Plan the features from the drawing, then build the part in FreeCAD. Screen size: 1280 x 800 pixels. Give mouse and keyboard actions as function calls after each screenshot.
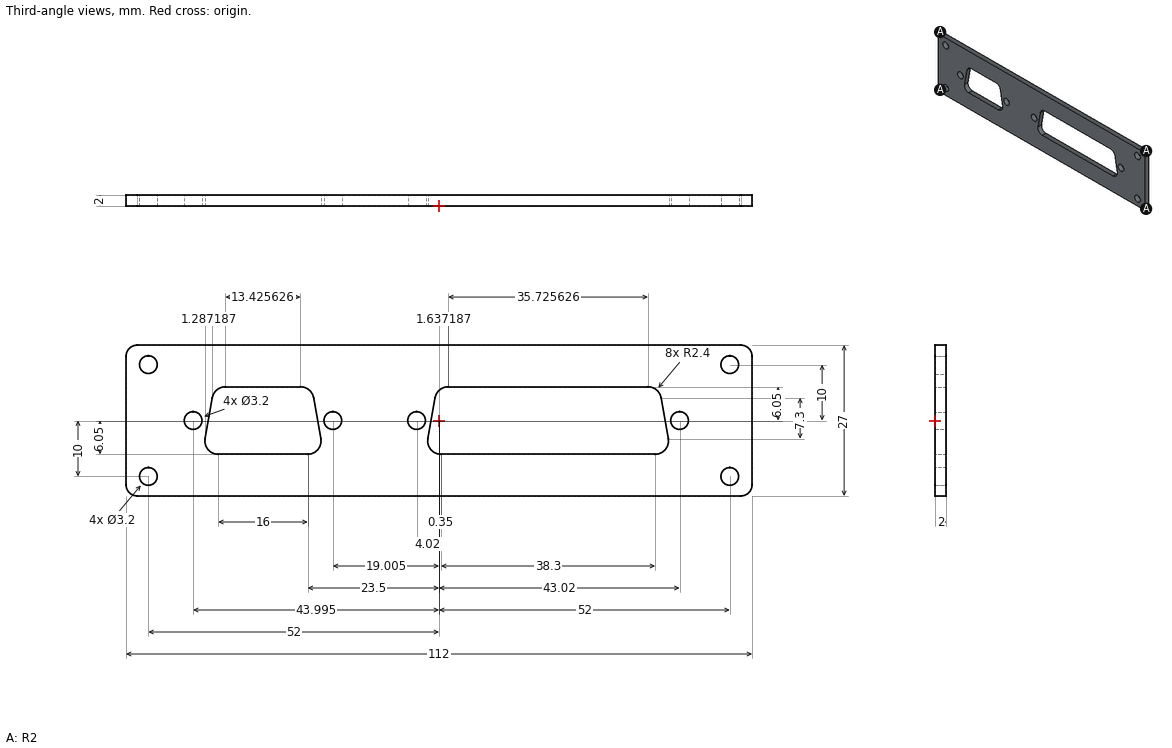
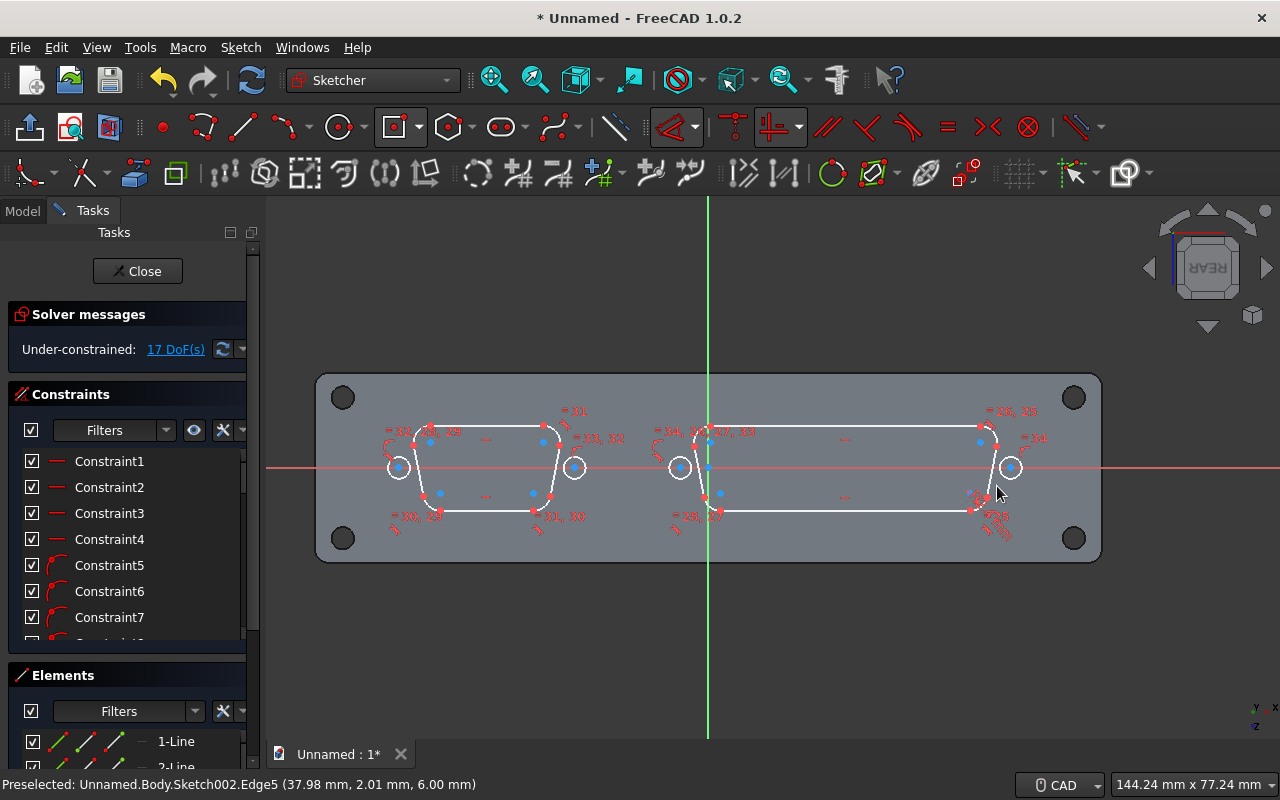
scroll(407, 460, up, 3)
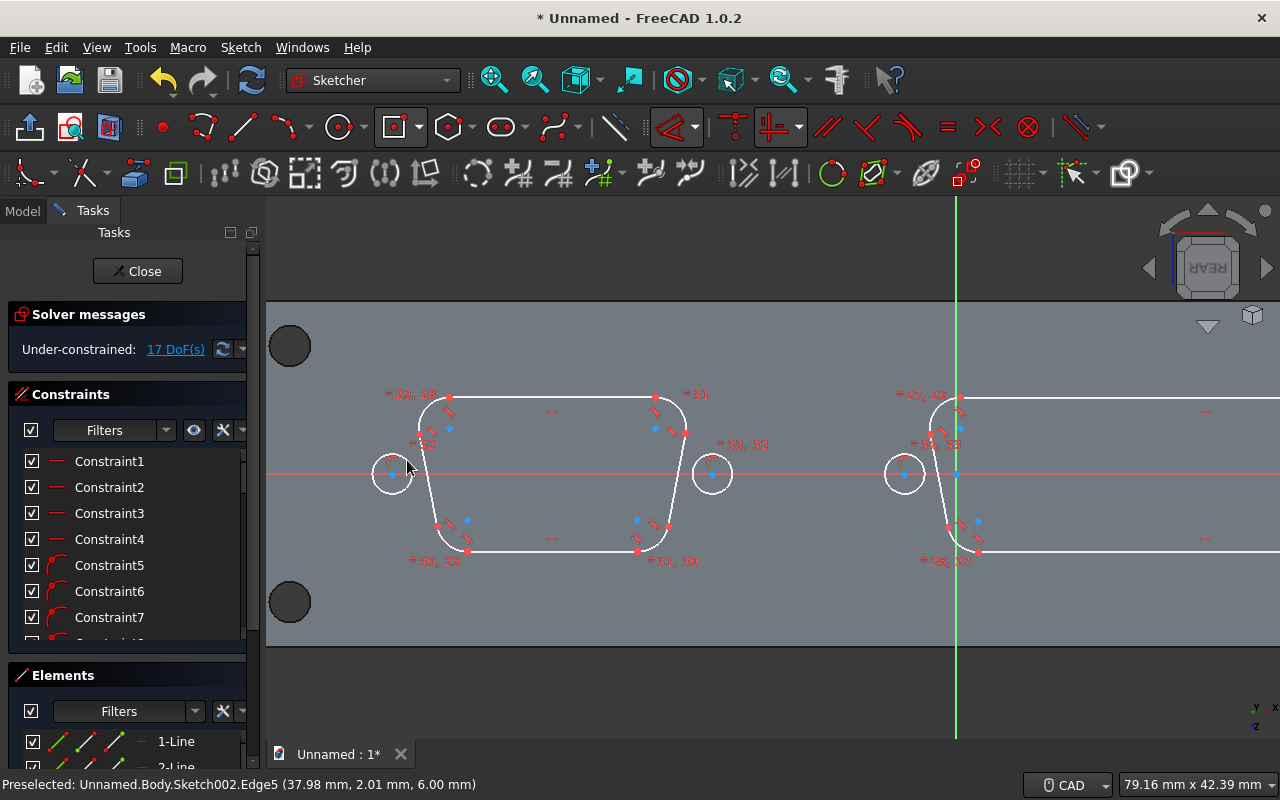
click(406, 460)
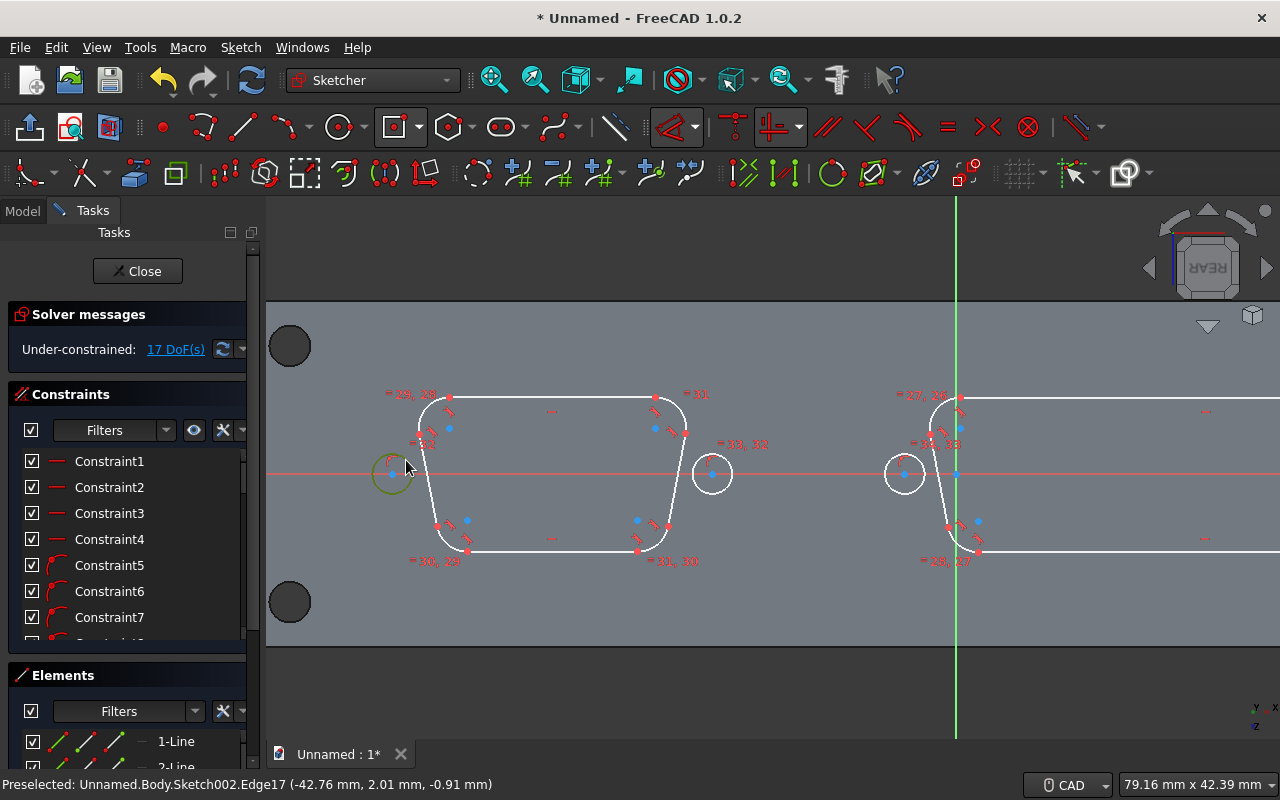
key(k)
key(o)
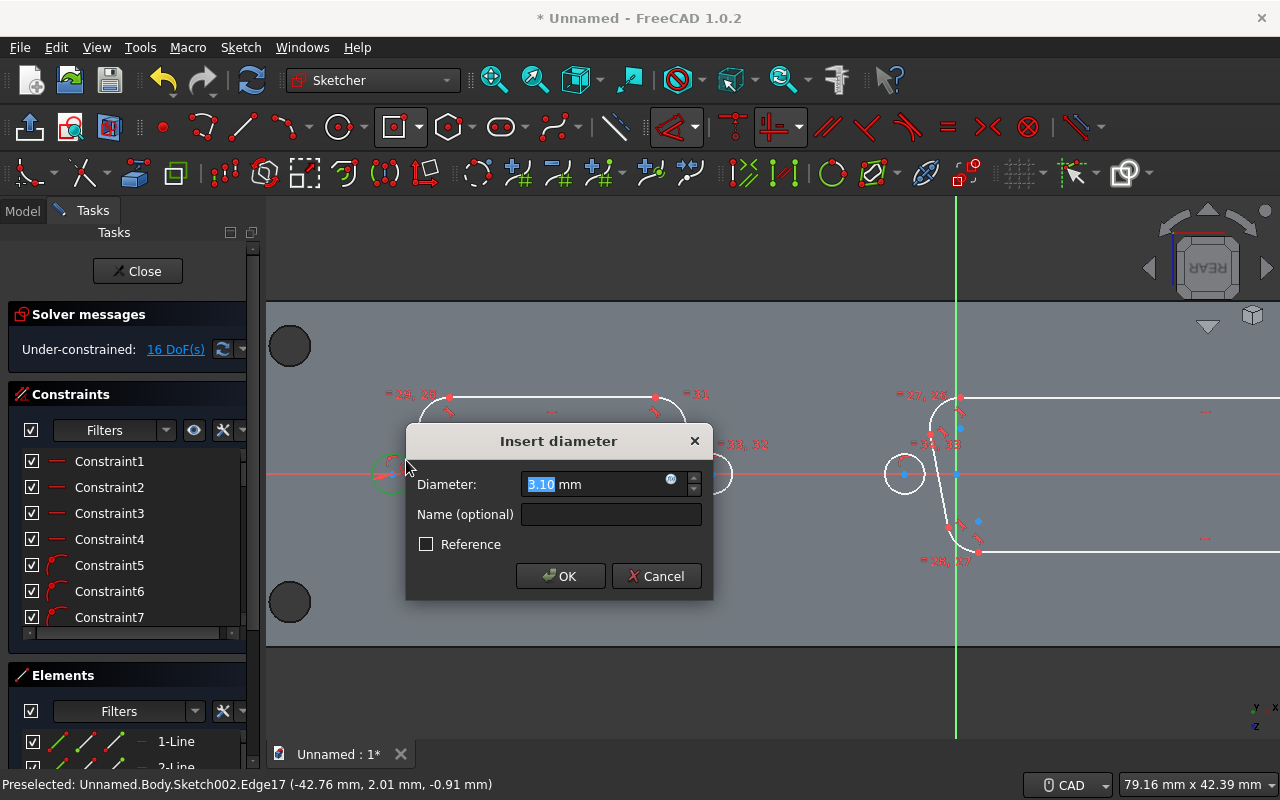
text(3.2)
key(Return)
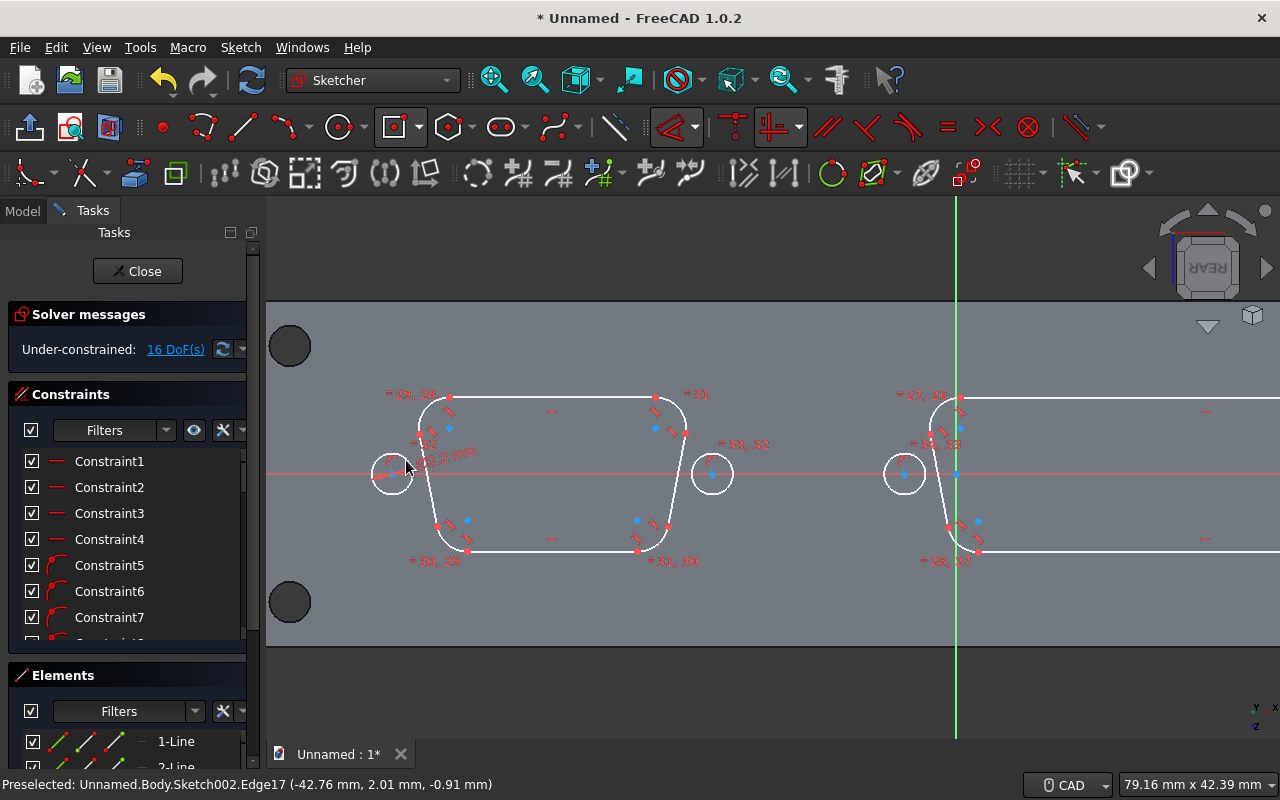
click(594, 397)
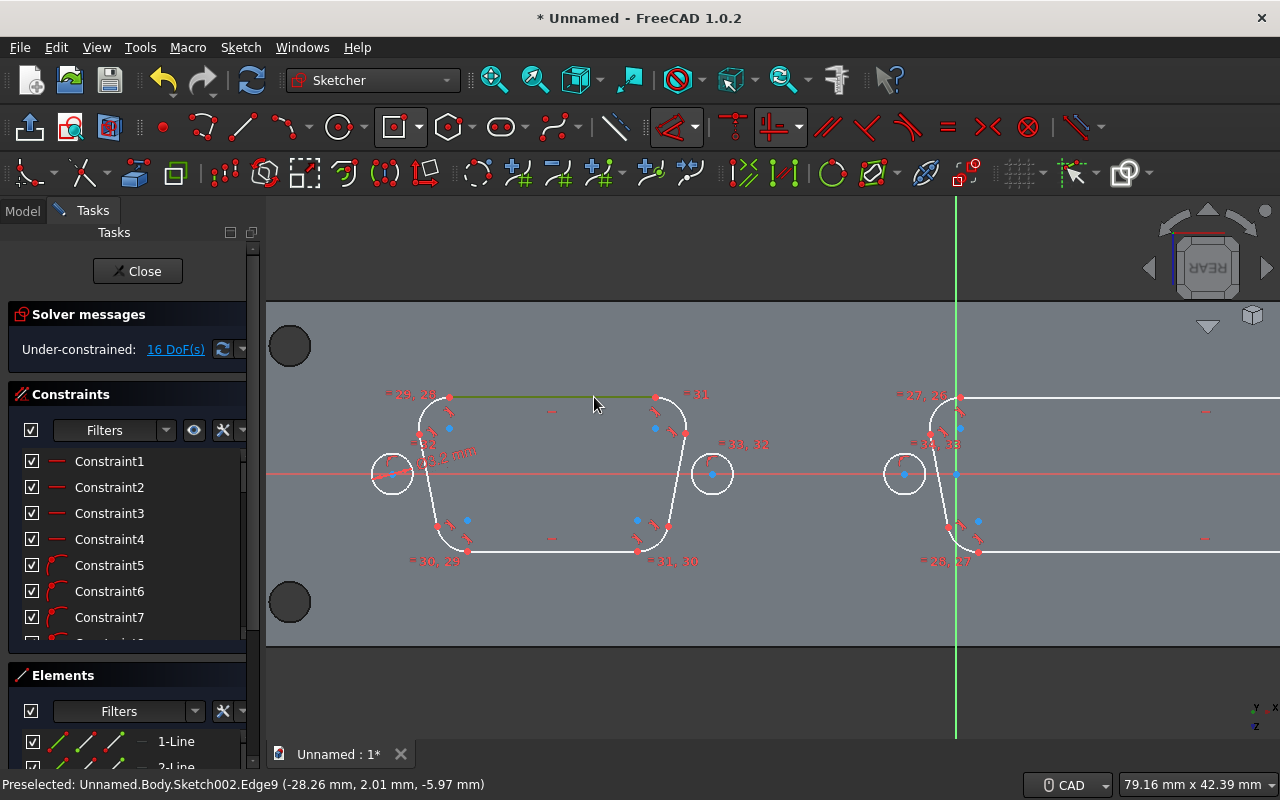
click(698, 128)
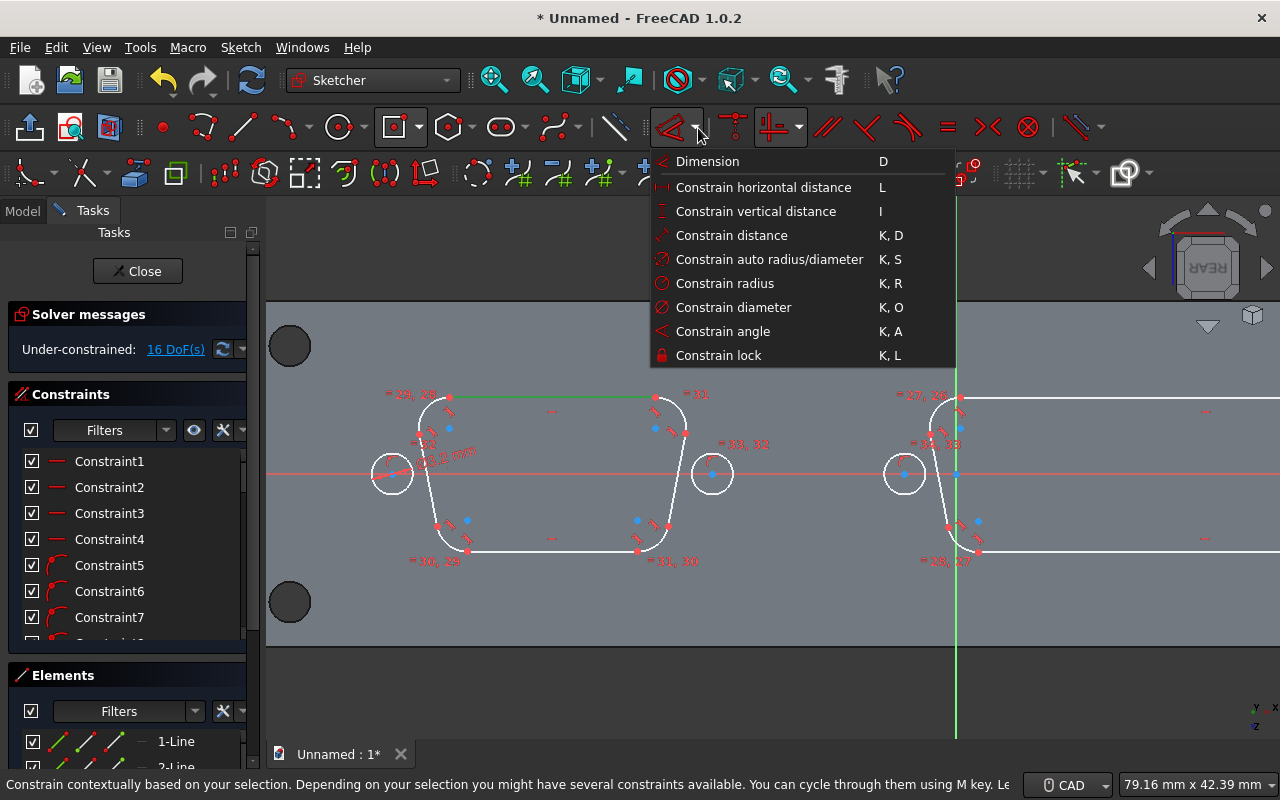
click(803, 187)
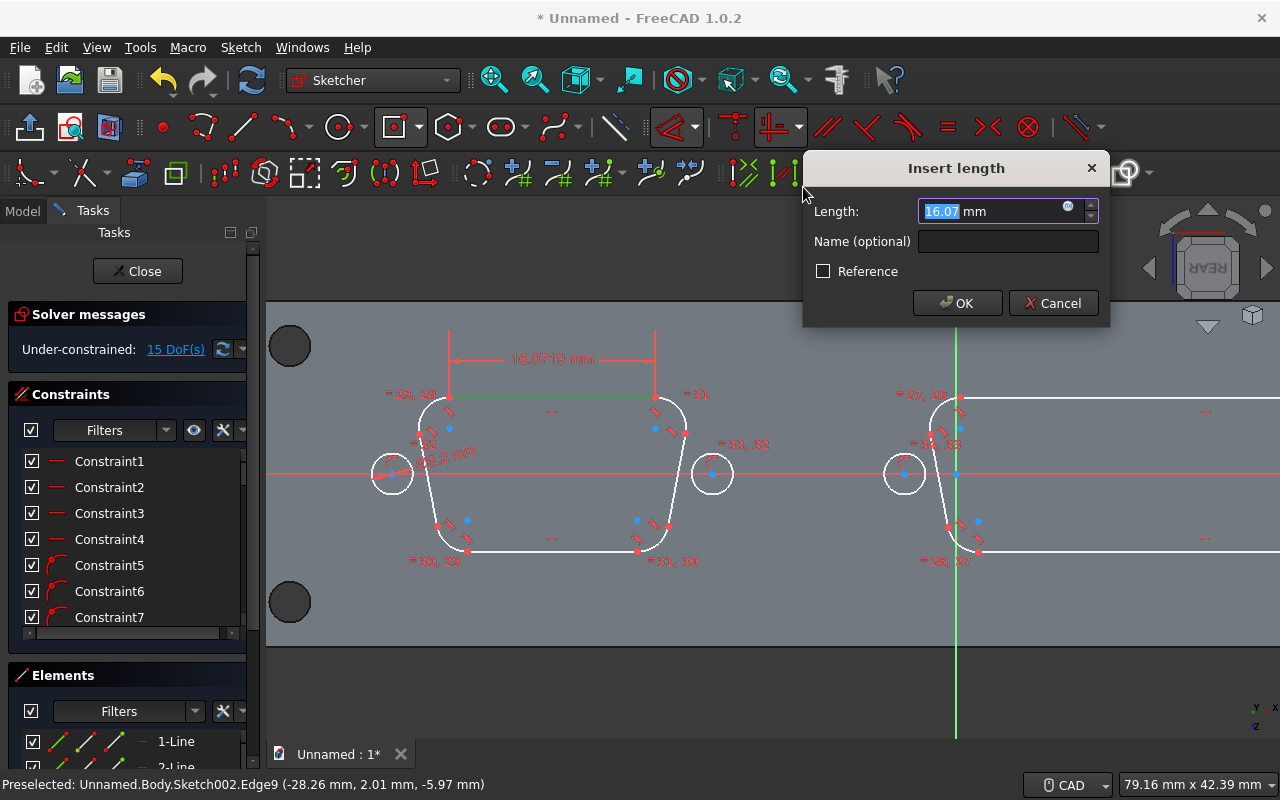
text(16)
key(Return)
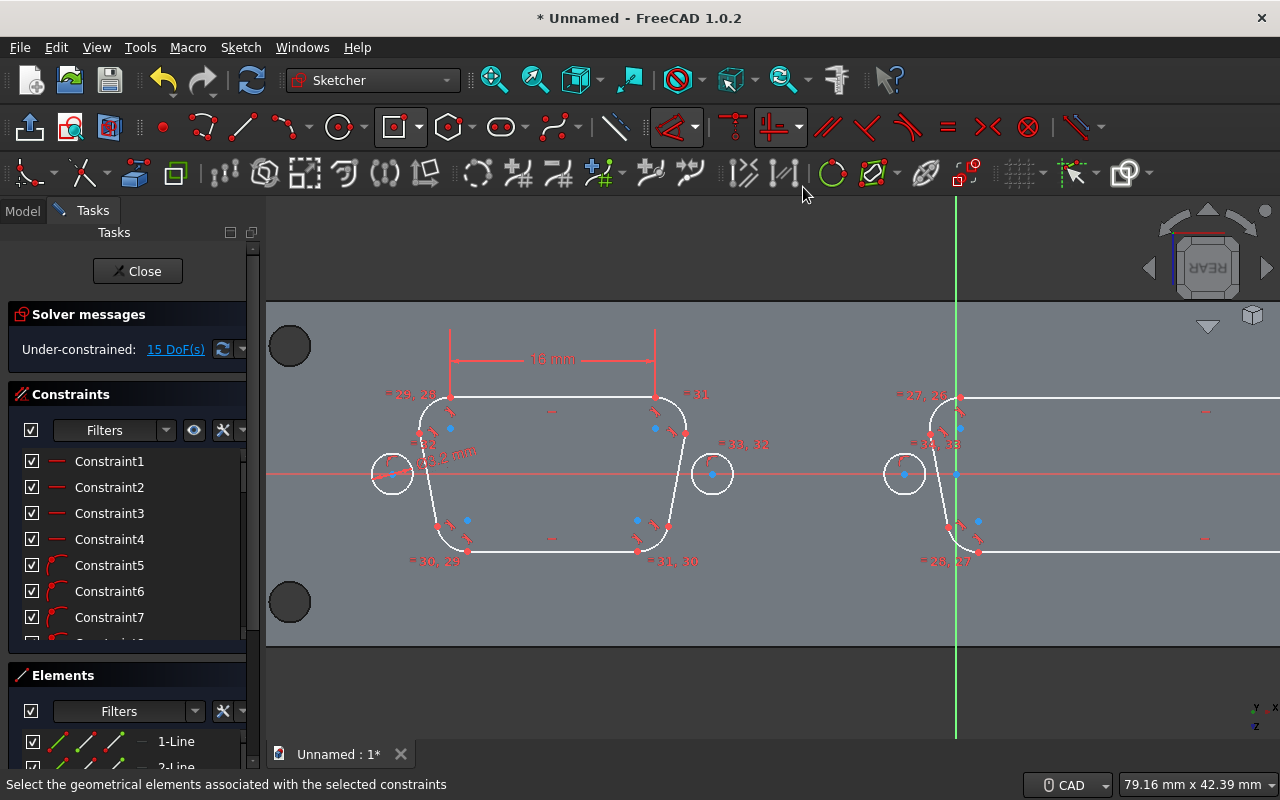
click(1108, 398)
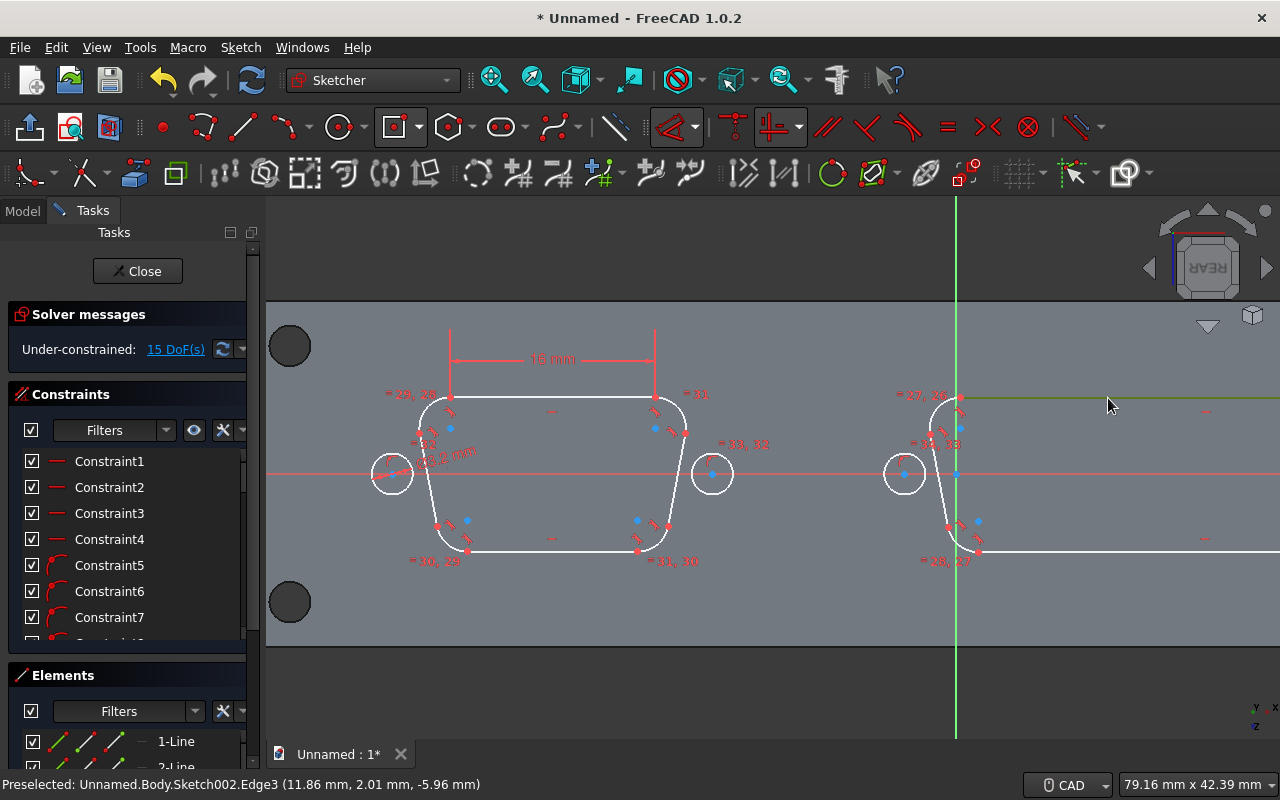
key(l)